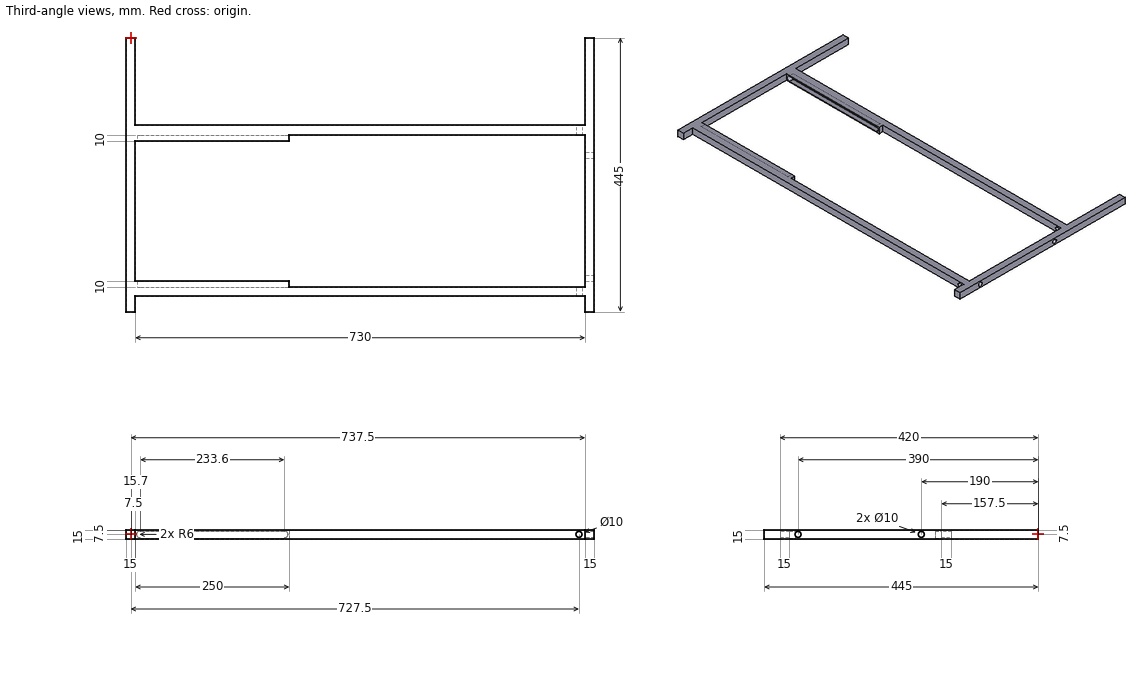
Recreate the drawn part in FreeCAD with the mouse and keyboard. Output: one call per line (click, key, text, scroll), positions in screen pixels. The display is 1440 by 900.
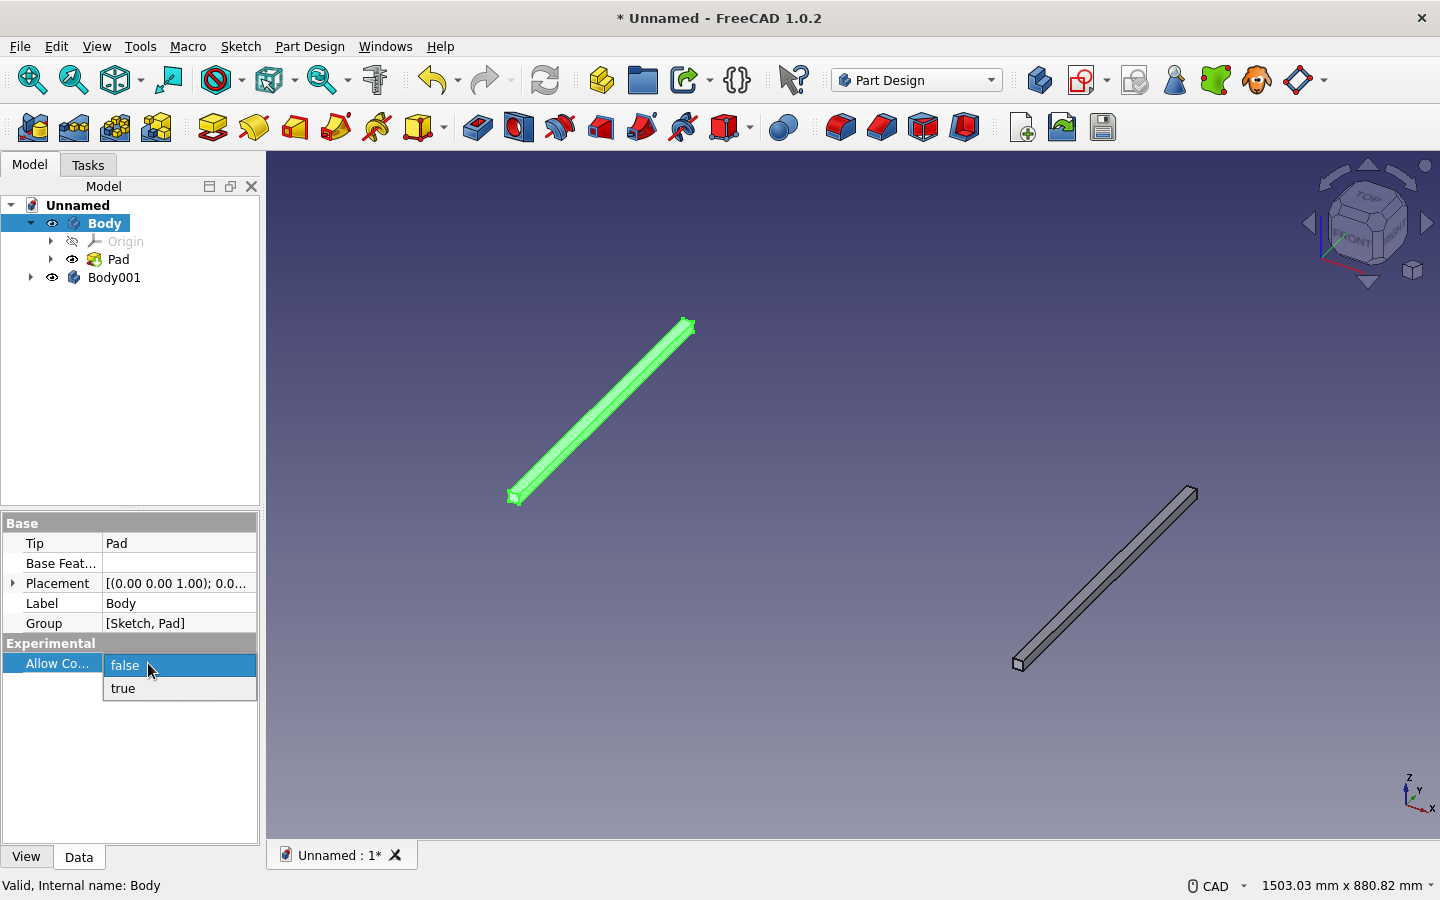
click(178, 688)
key(Return)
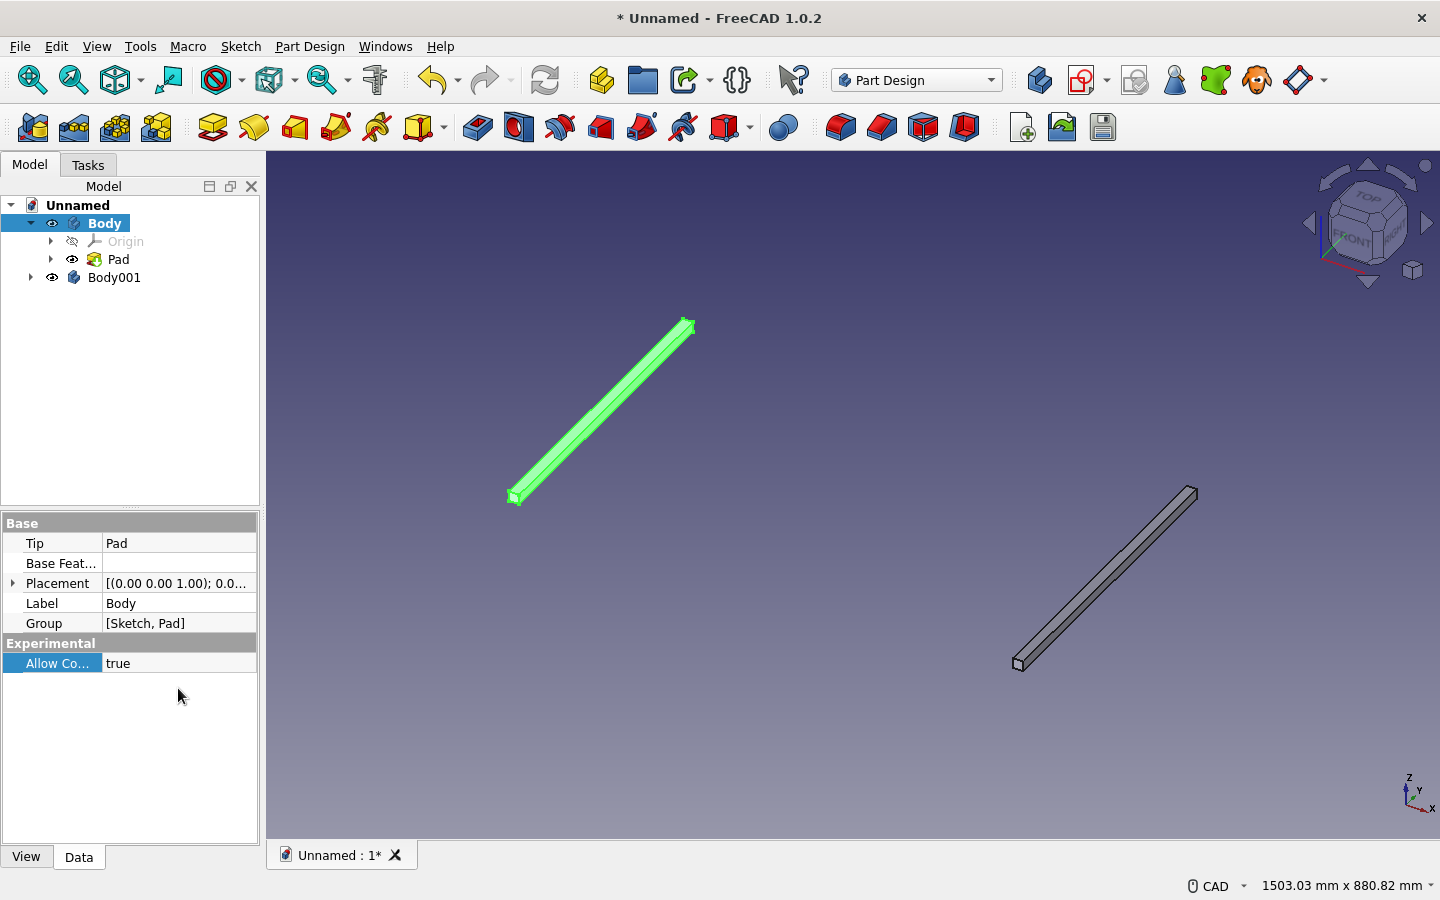
click(97, 277)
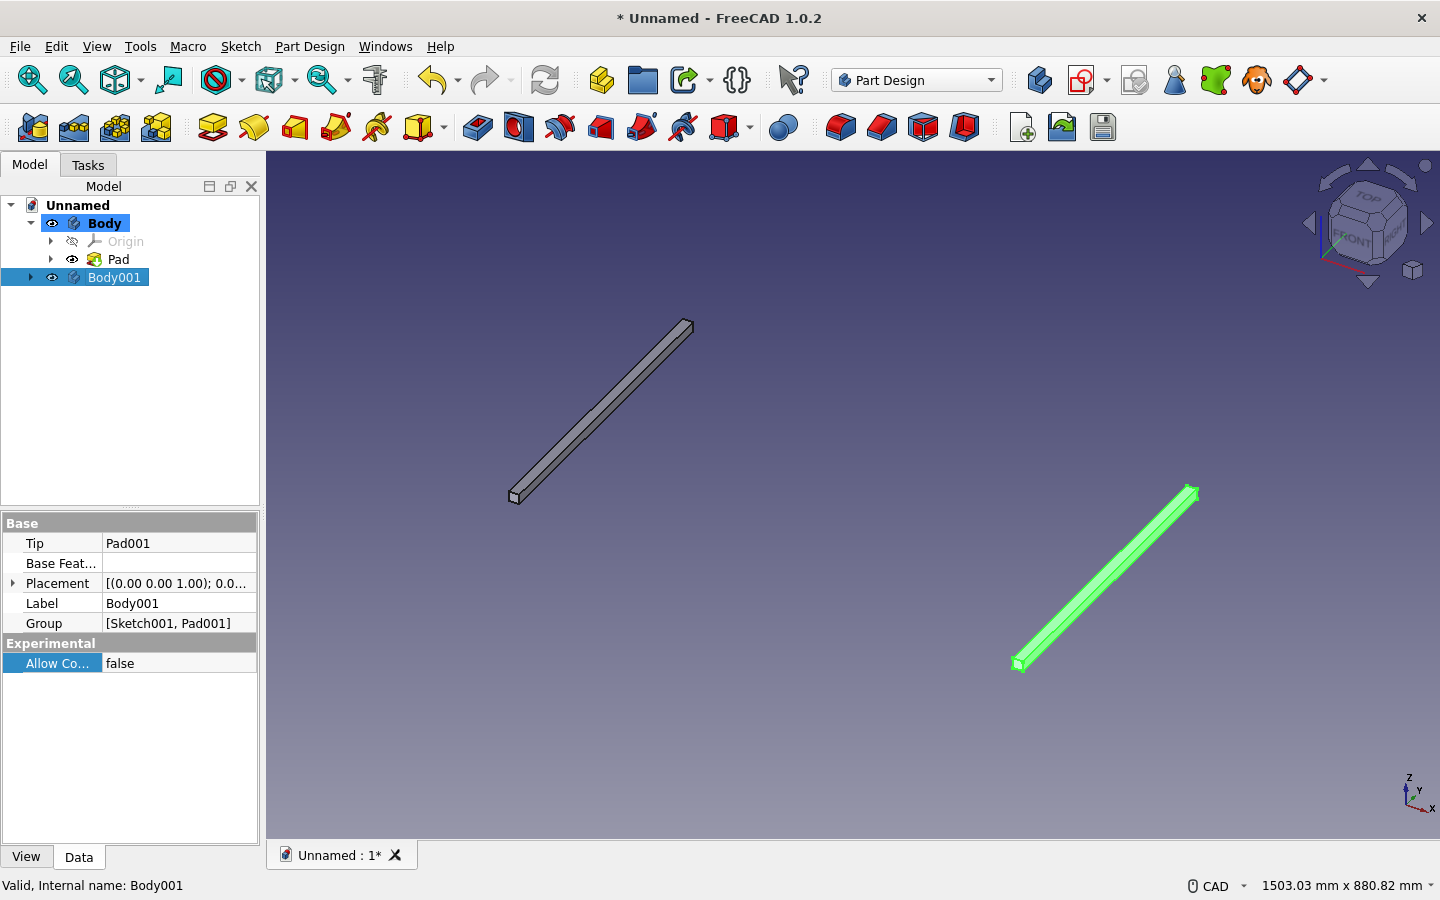
click(784, 128)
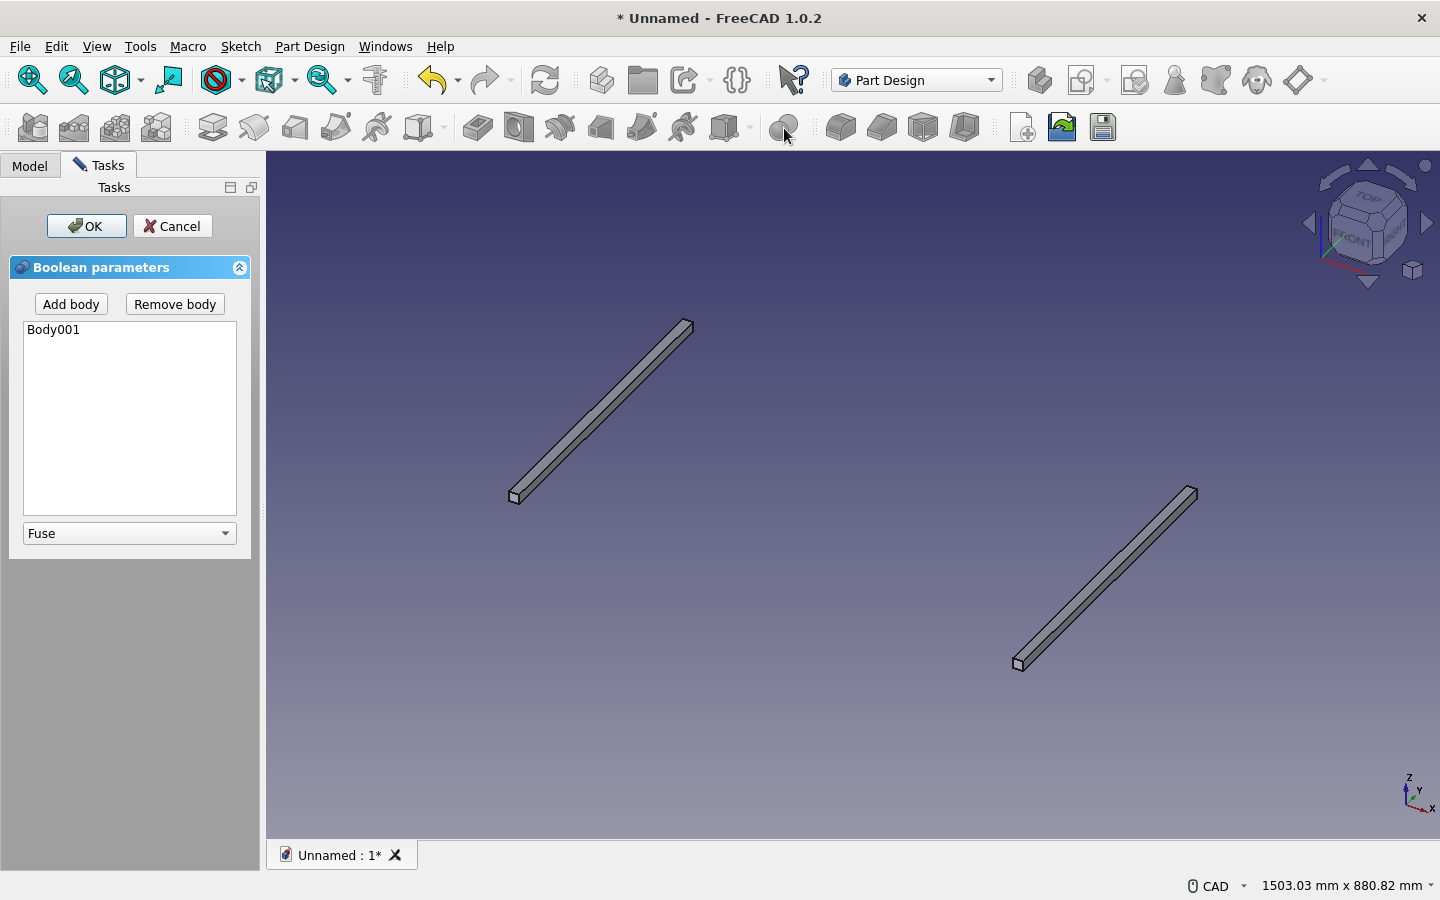
click(87, 226)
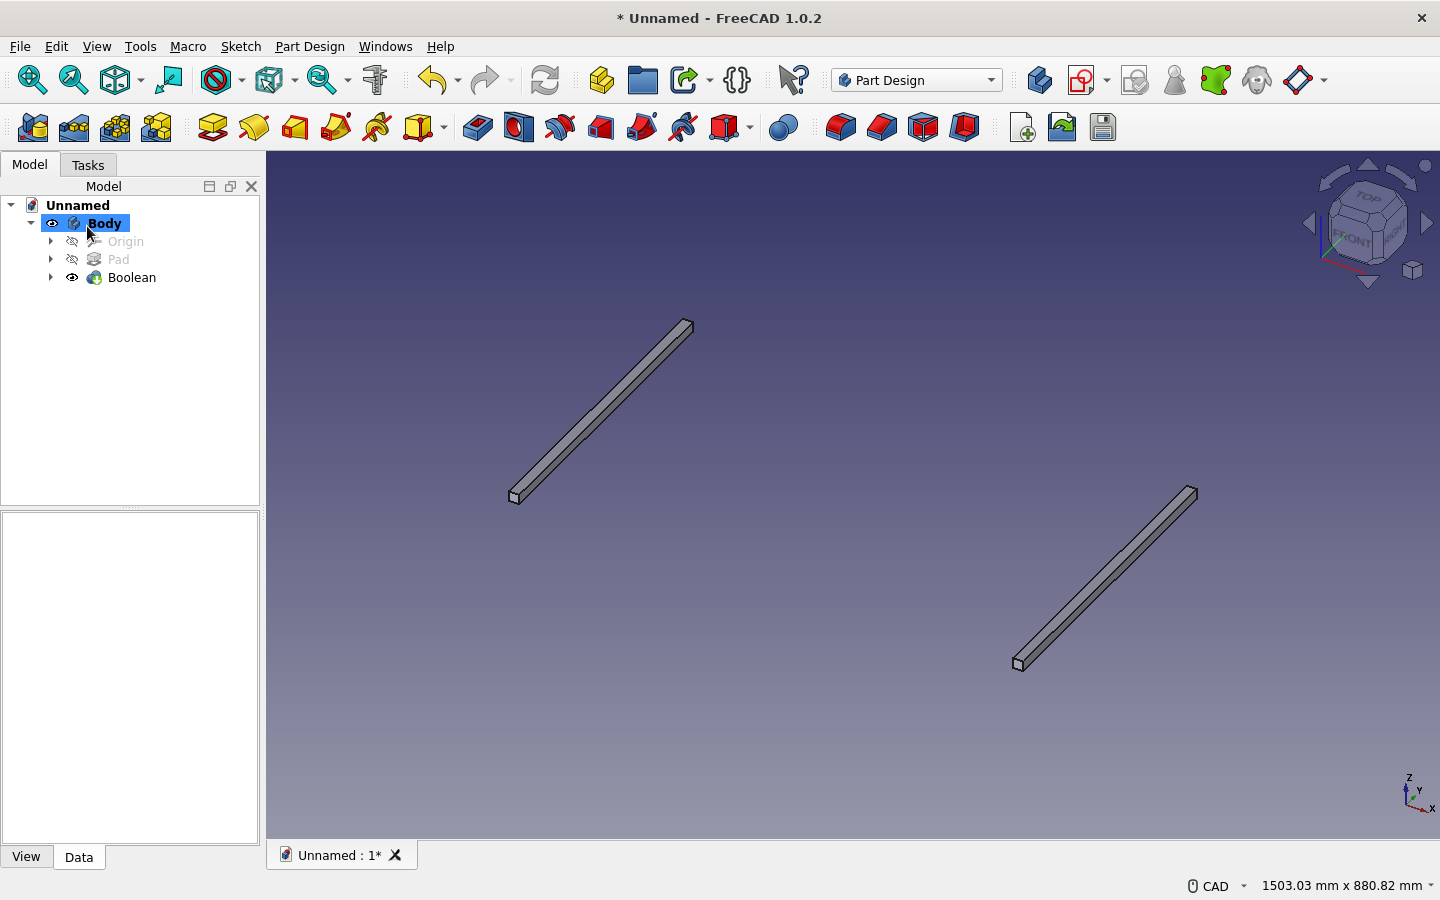
click(51, 241)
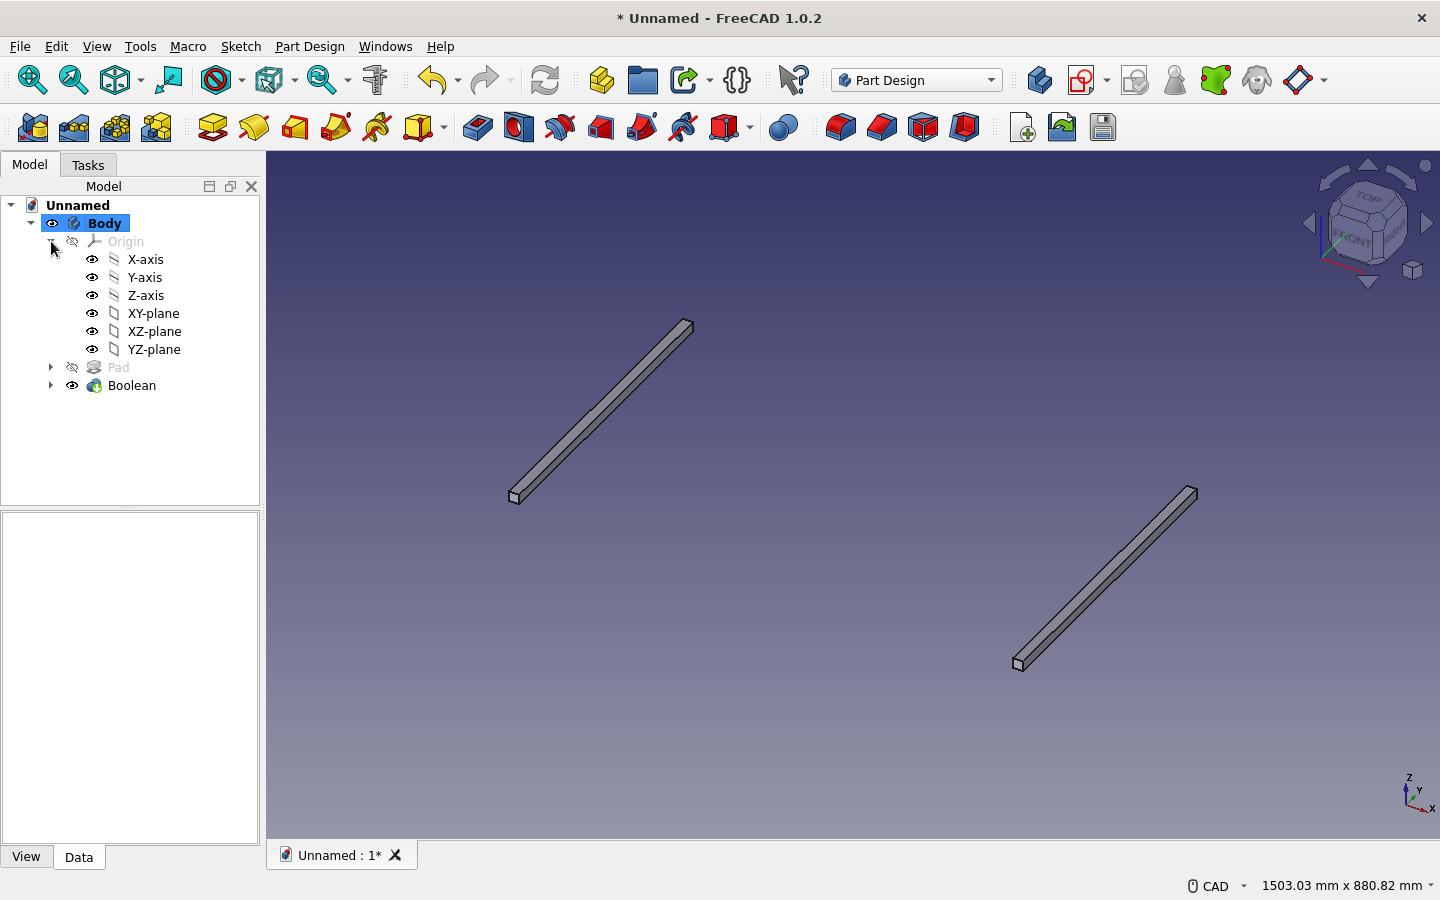
click(137, 349)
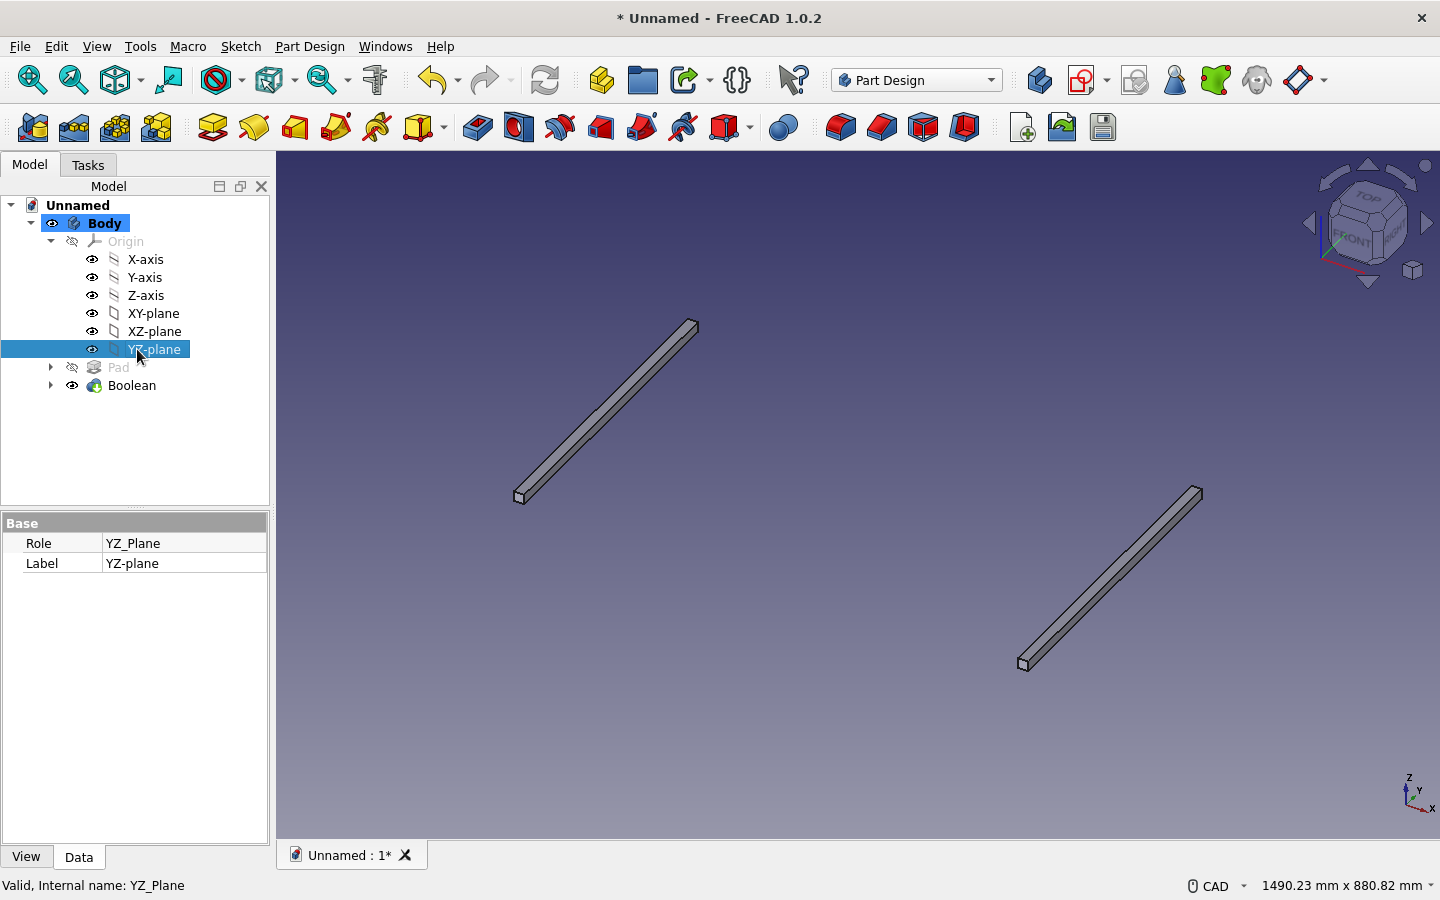
click(1298, 80)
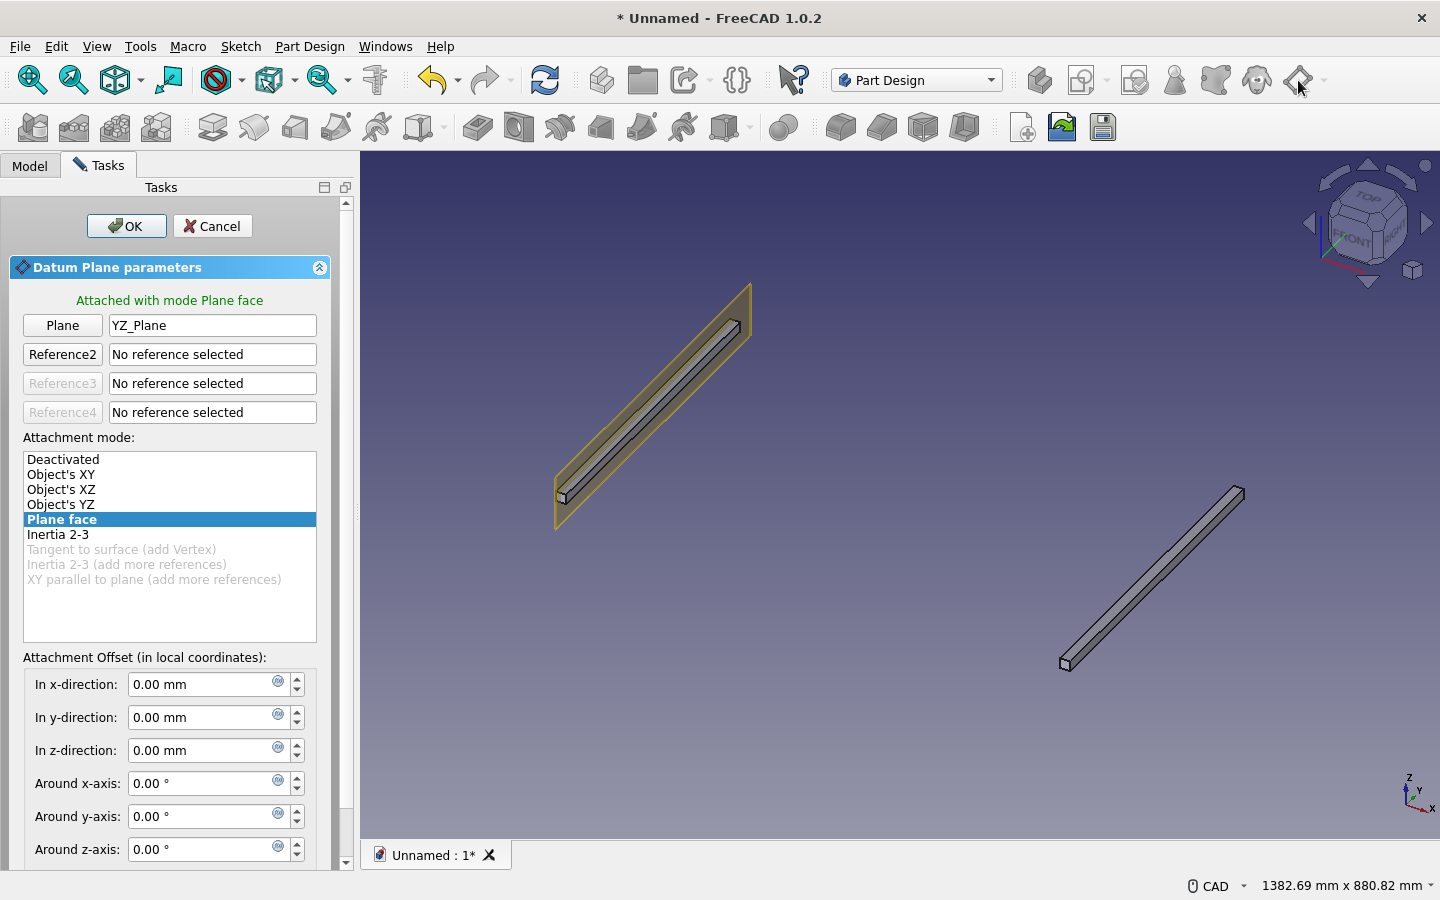
triple_click(210, 750)